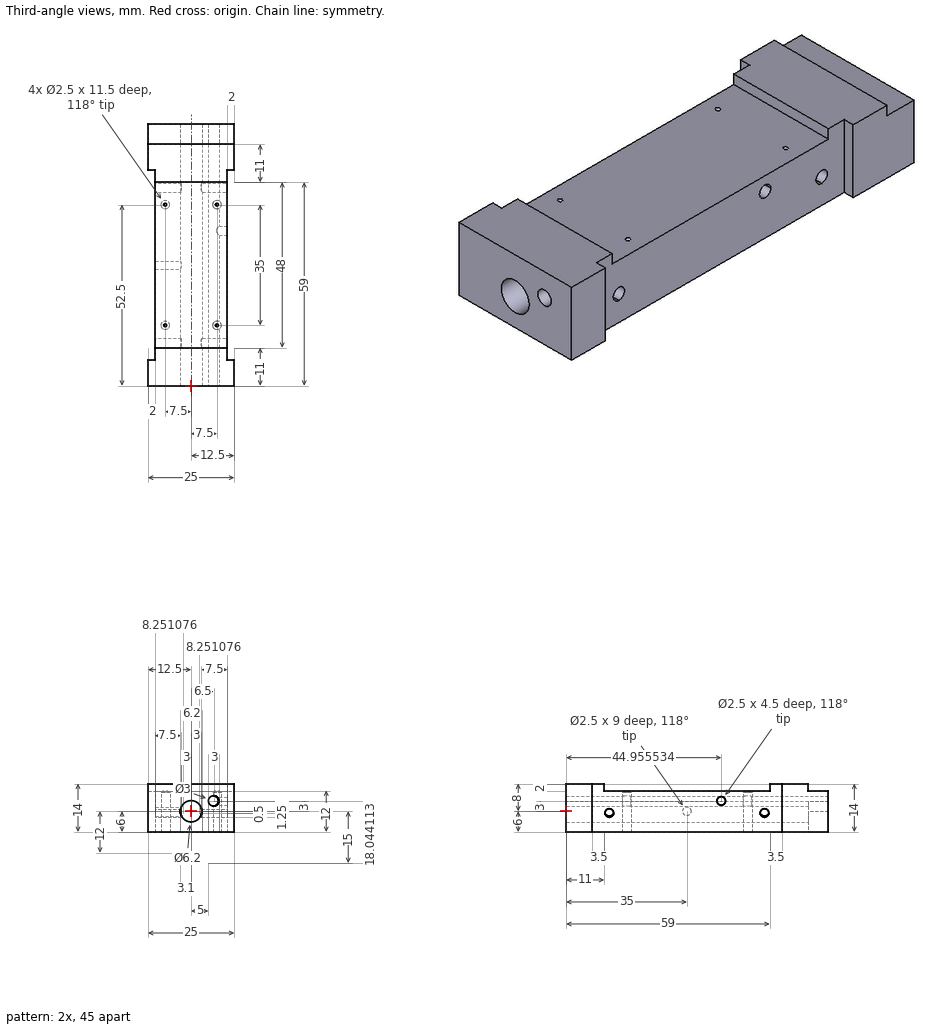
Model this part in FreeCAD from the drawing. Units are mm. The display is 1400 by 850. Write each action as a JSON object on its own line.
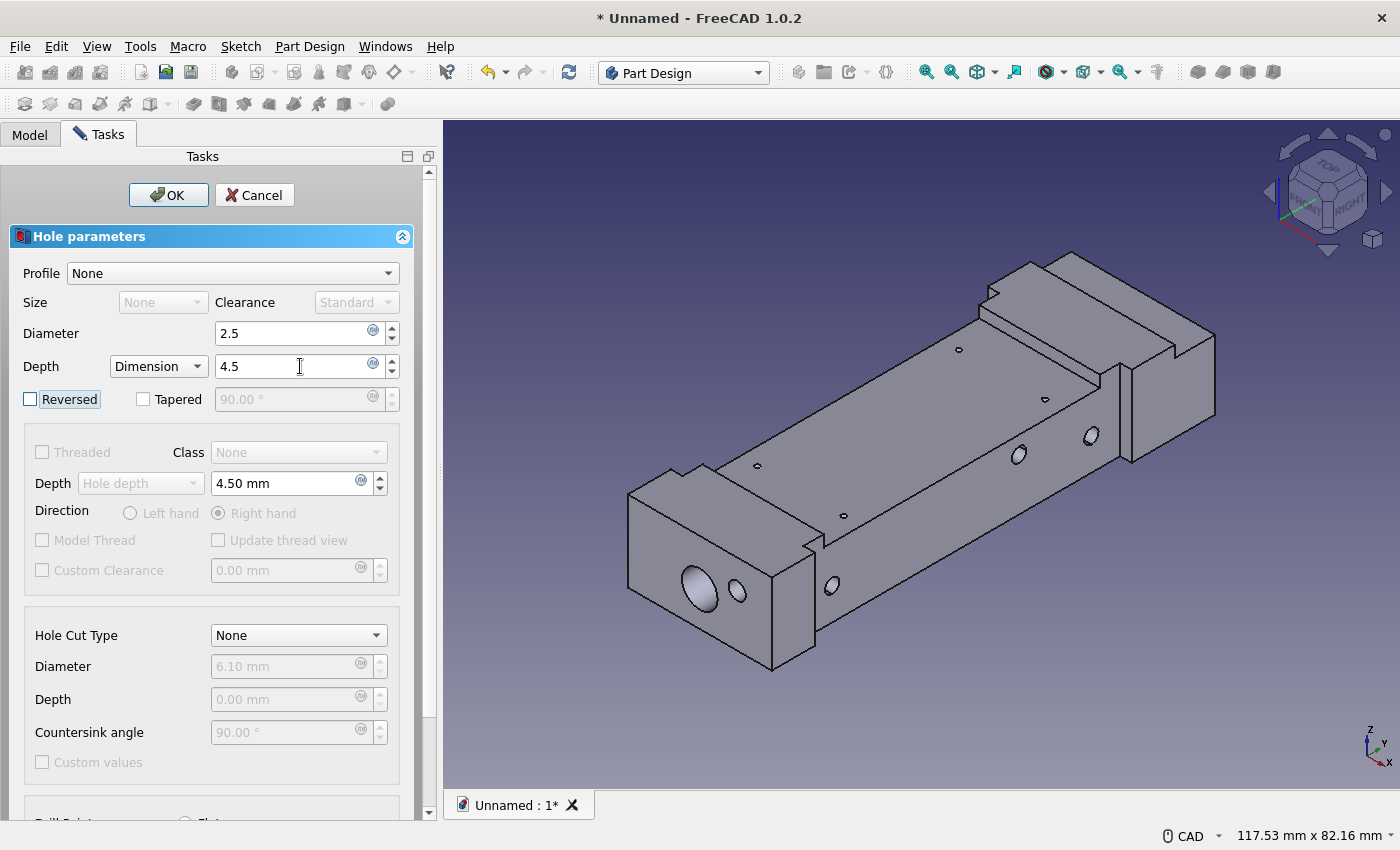
{"action": "left_click", "coordinate": [169, 195]}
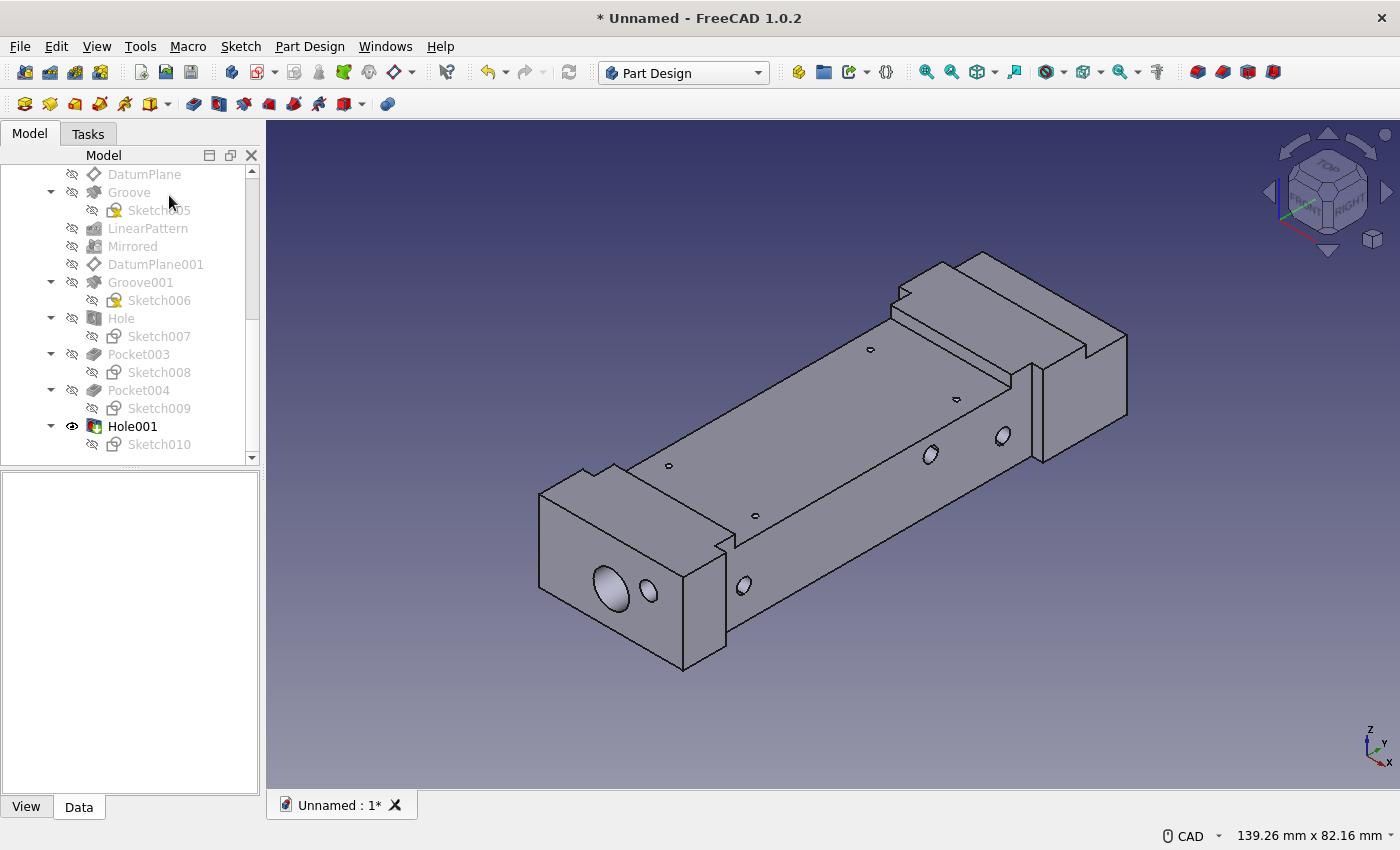
{"action": "key", "text": "4"}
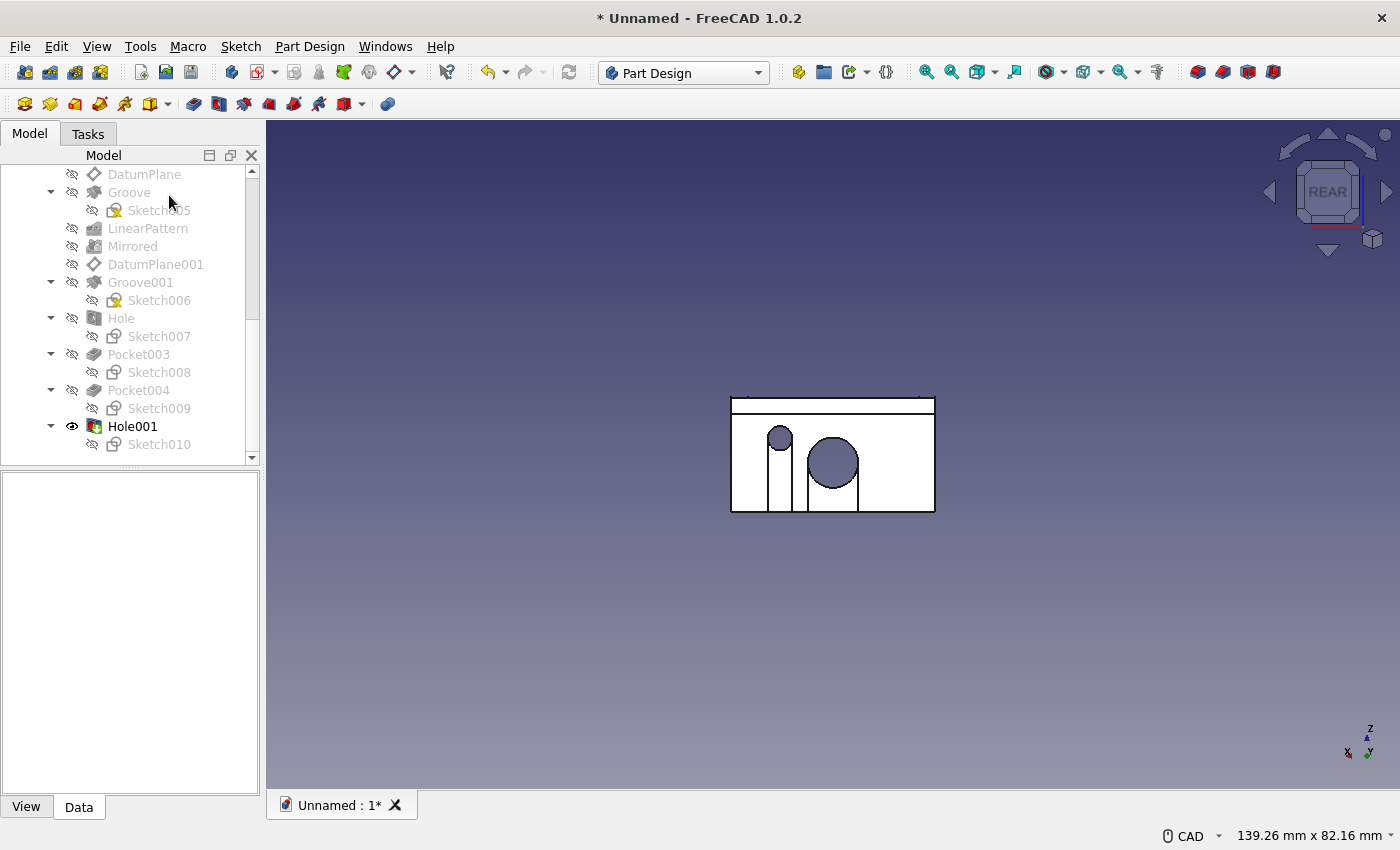
{"action": "left_click", "coordinate": [927, 72]}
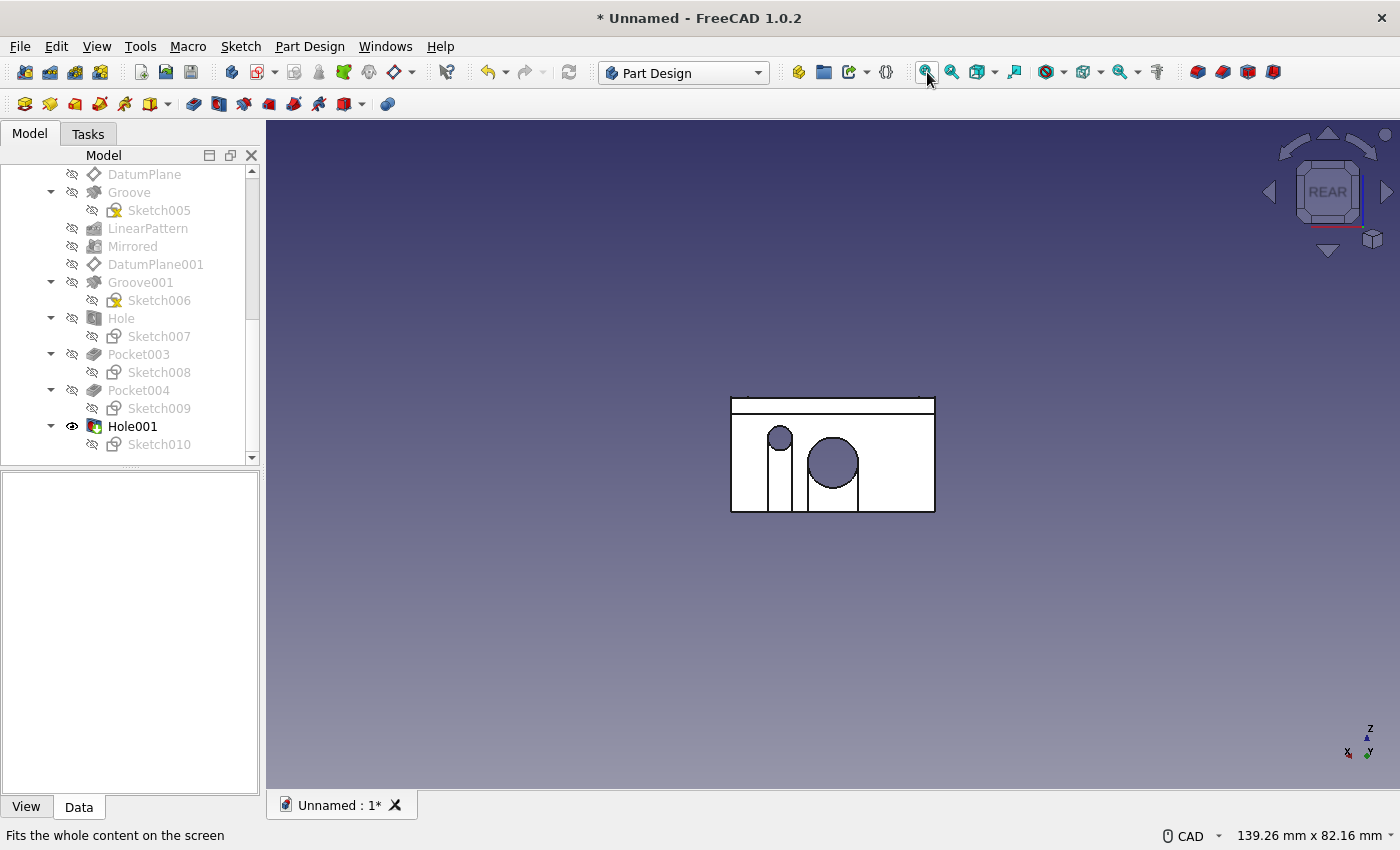
{"action": "left_click", "coordinate": [891, 448]}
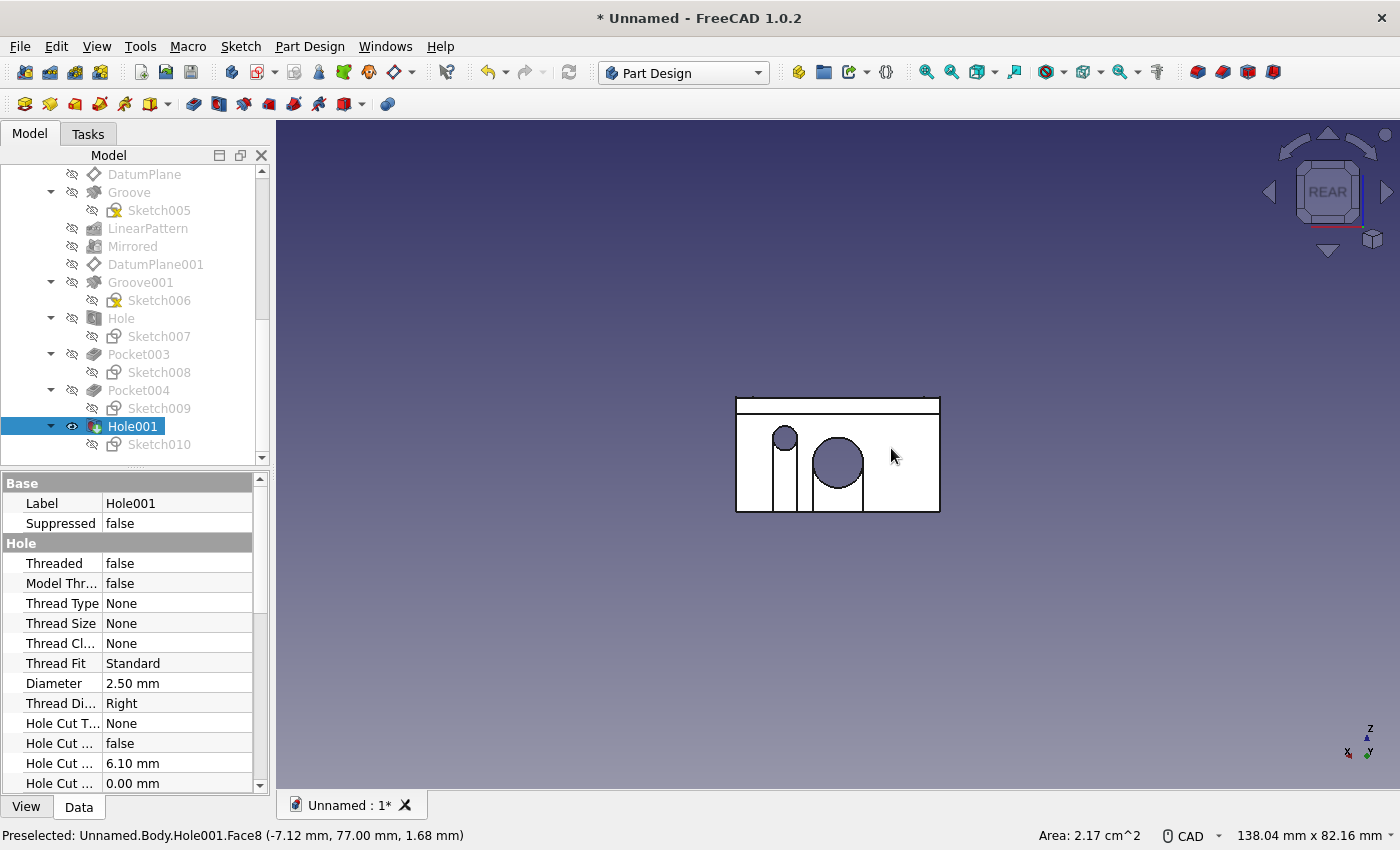
{"action": "left_click", "coordinate": [256, 72]}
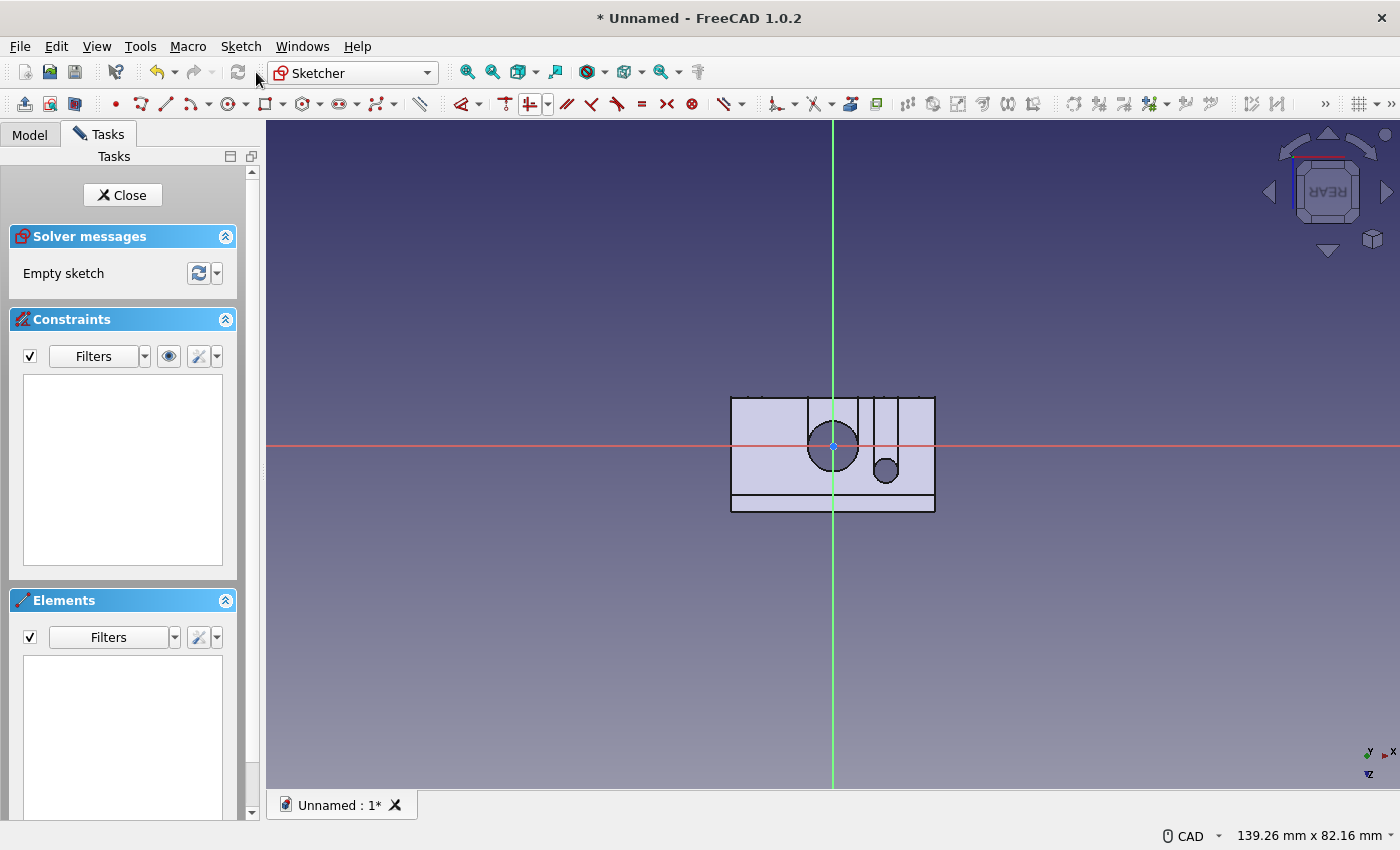
{"action": "scroll", "coordinate": [863, 454], "scroll_direction": "up", "scroll_amount": 6}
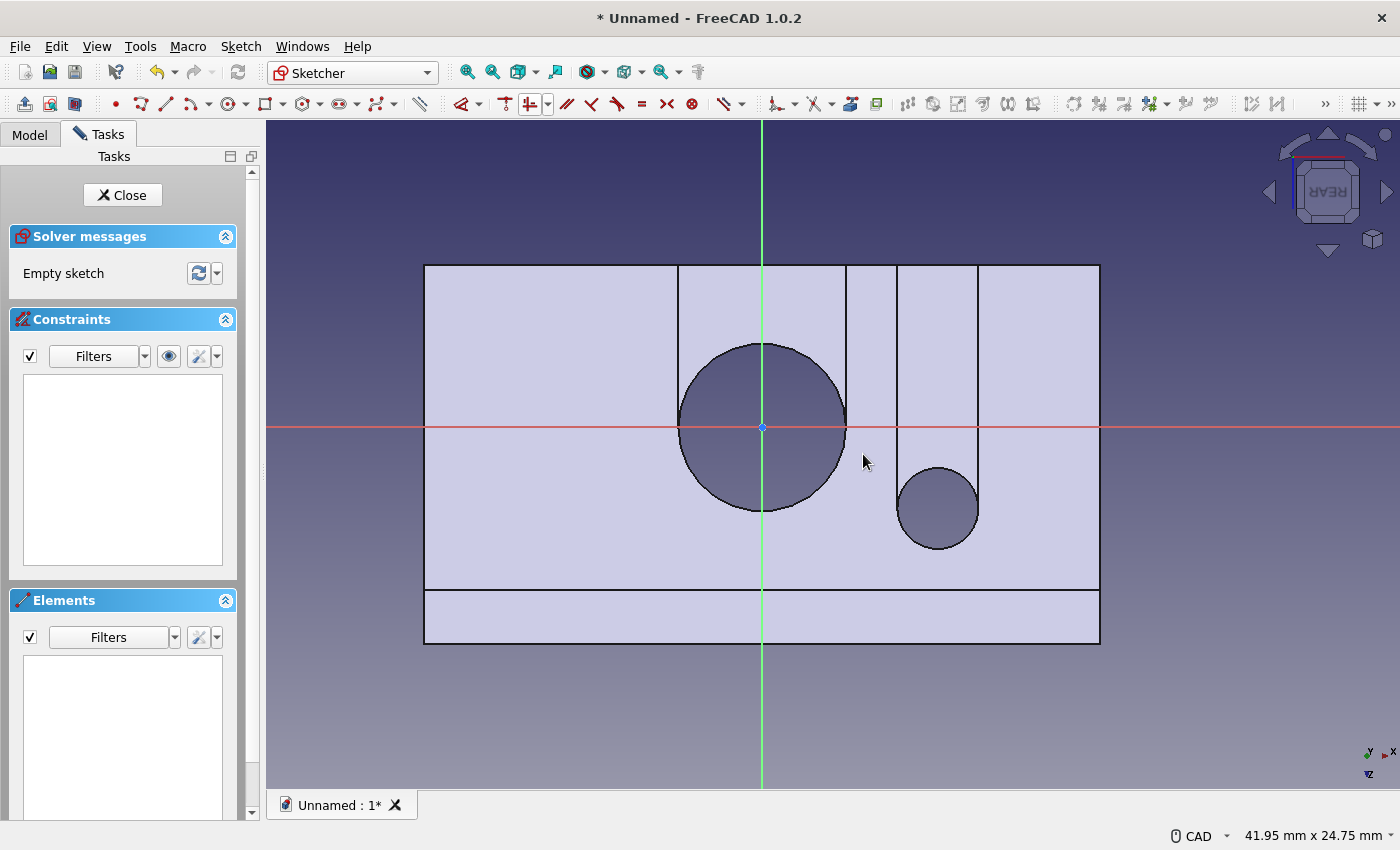
{"action": "left_click", "coordinate": [264, 104]}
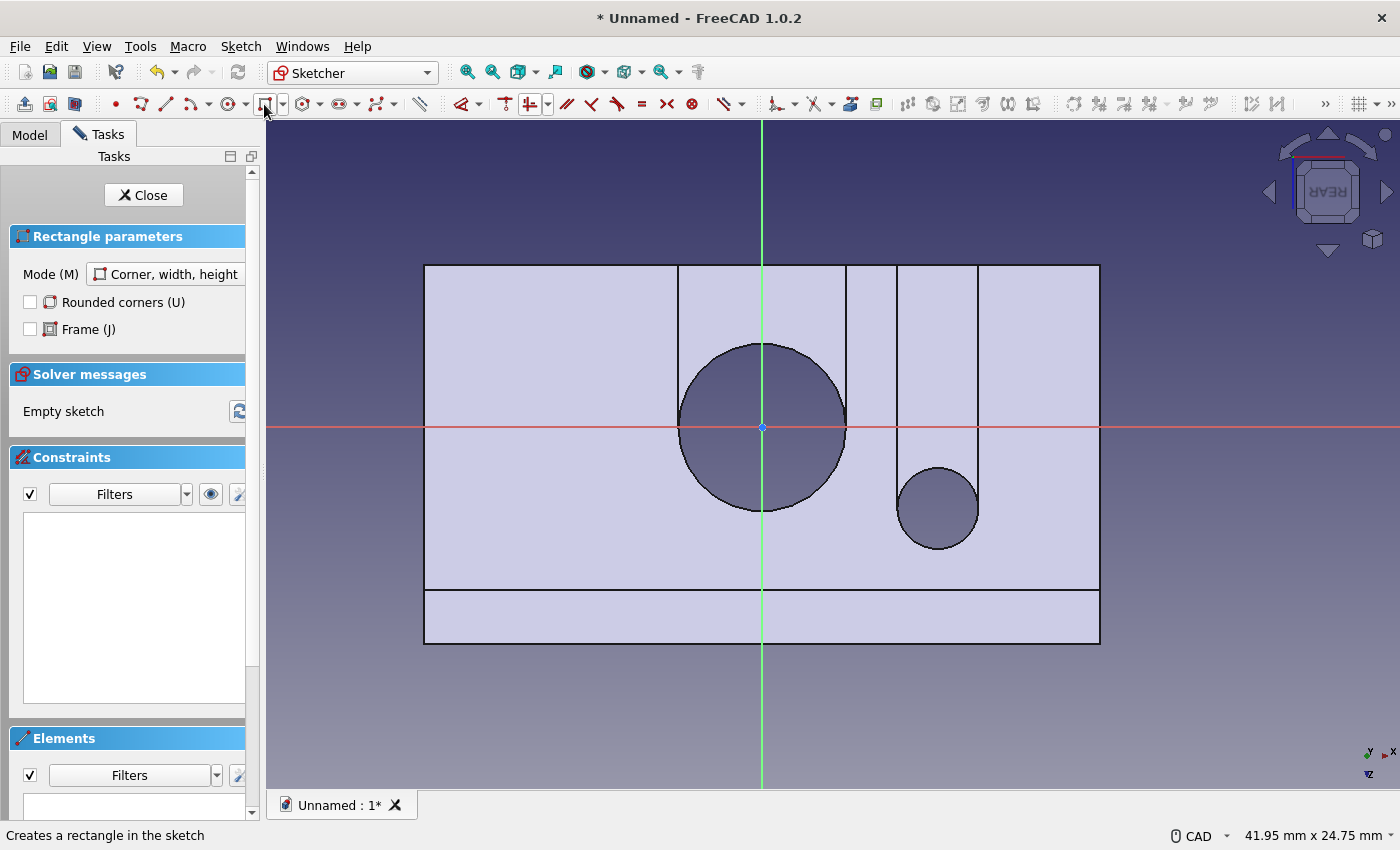
{"action": "left_click", "coordinate": [424, 265]}
{"action": "left_click", "coordinate": [1100, 644]}
{"action": "key", "text": "Escape"}